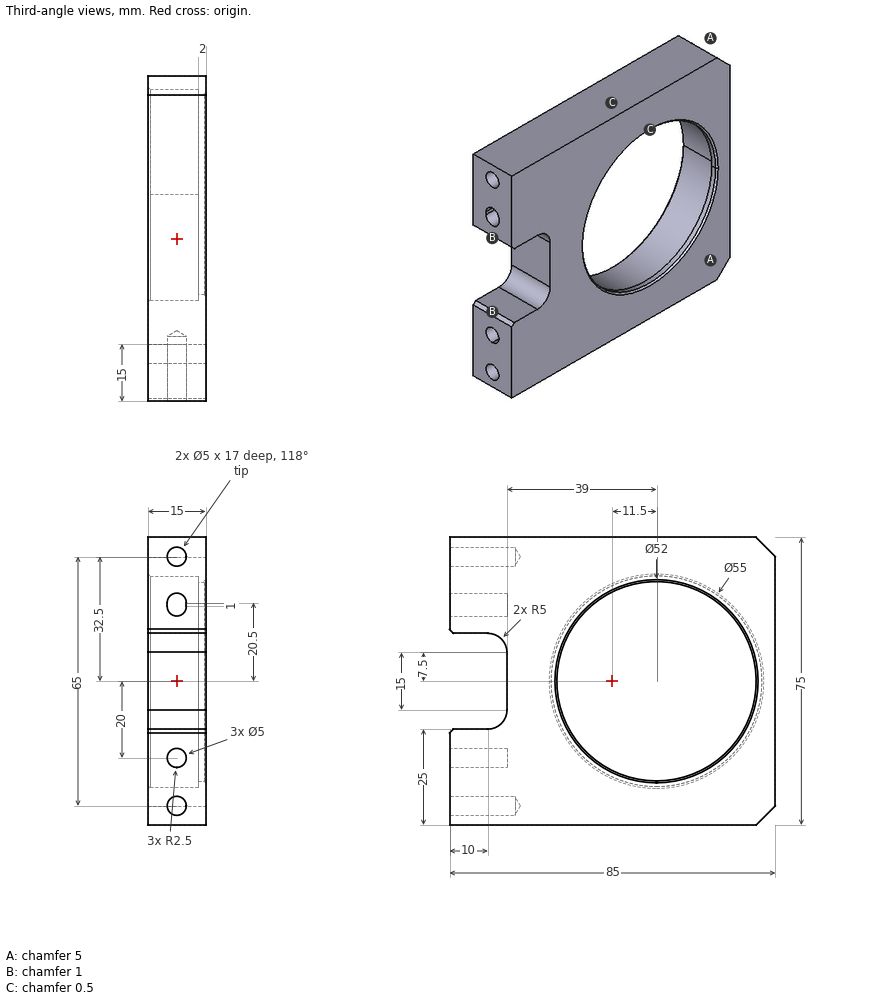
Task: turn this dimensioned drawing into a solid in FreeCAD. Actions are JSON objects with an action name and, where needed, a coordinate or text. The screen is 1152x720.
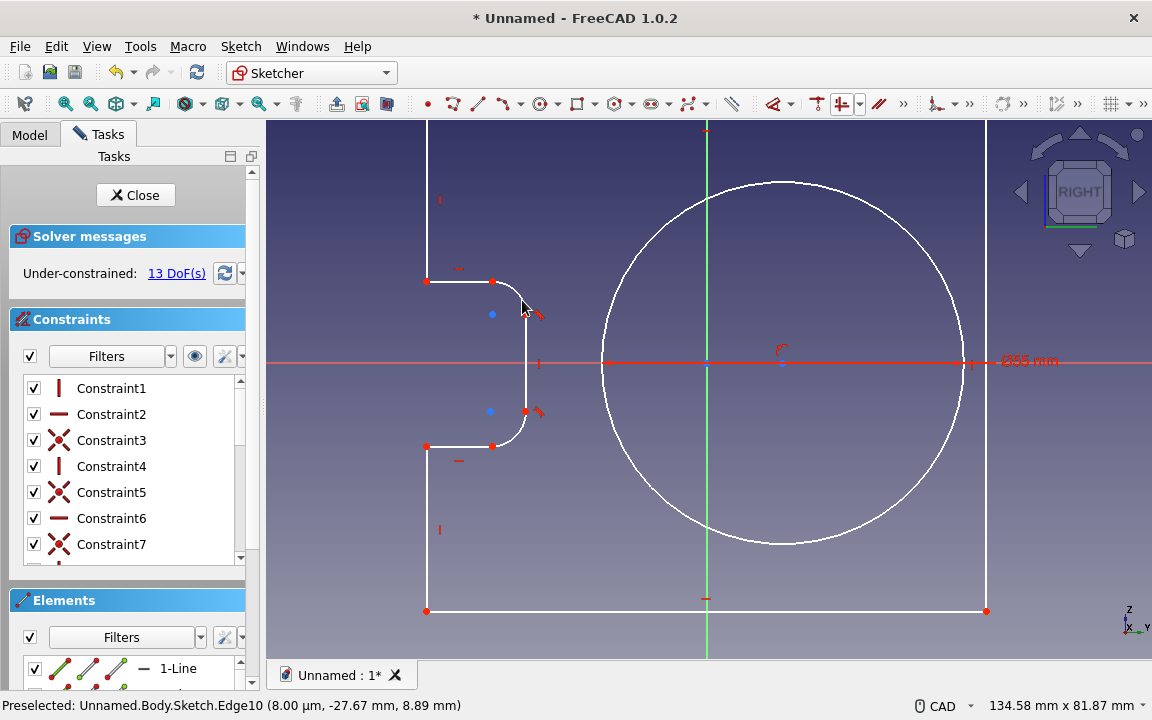
{"action": "left_click", "coordinate": [473, 447]}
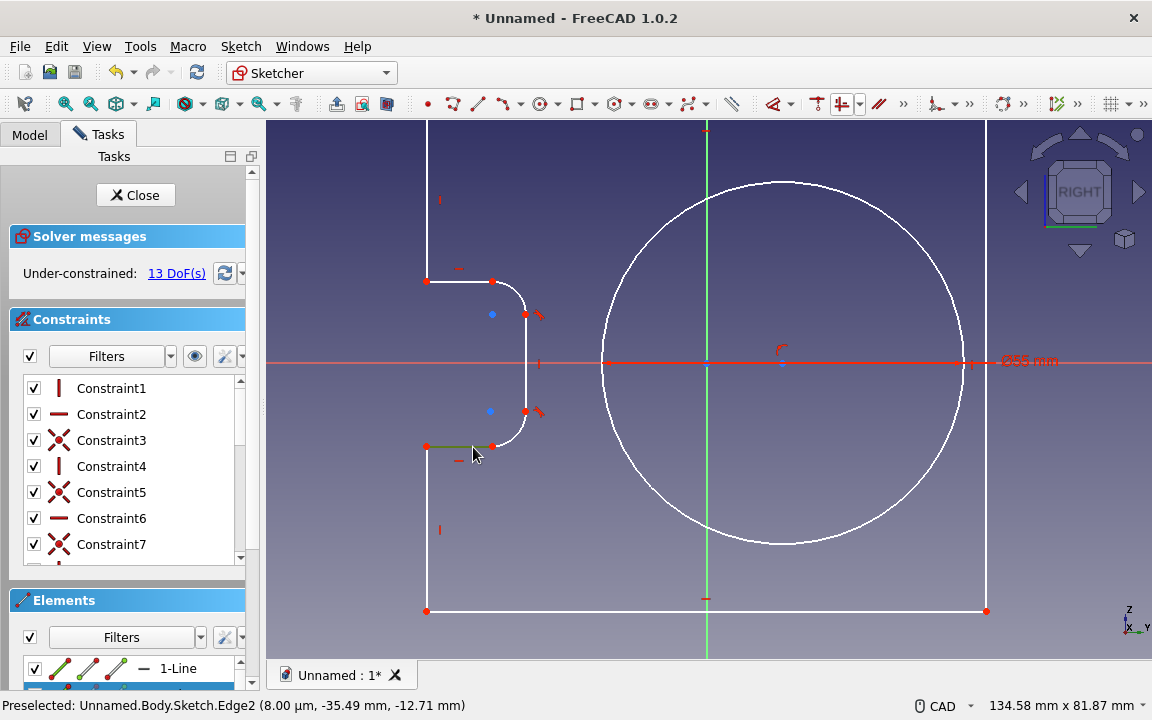
{"action": "left_click", "coordinate": [508, 442]}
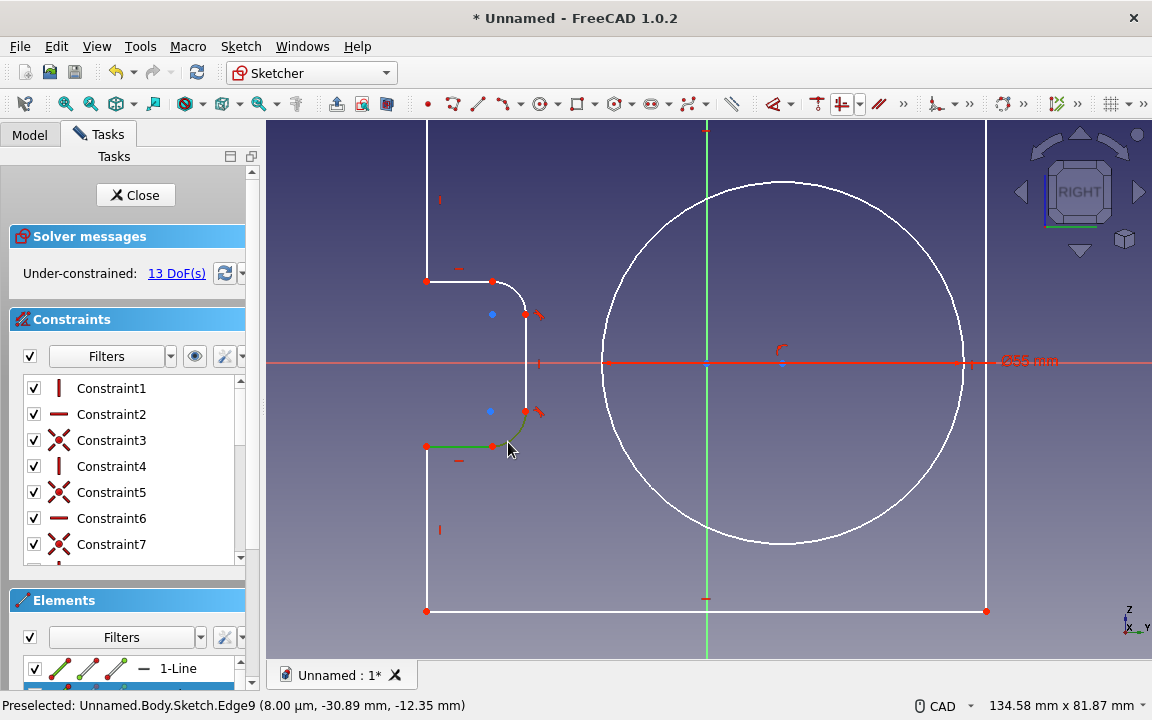
{"action": "key", "text": "t"}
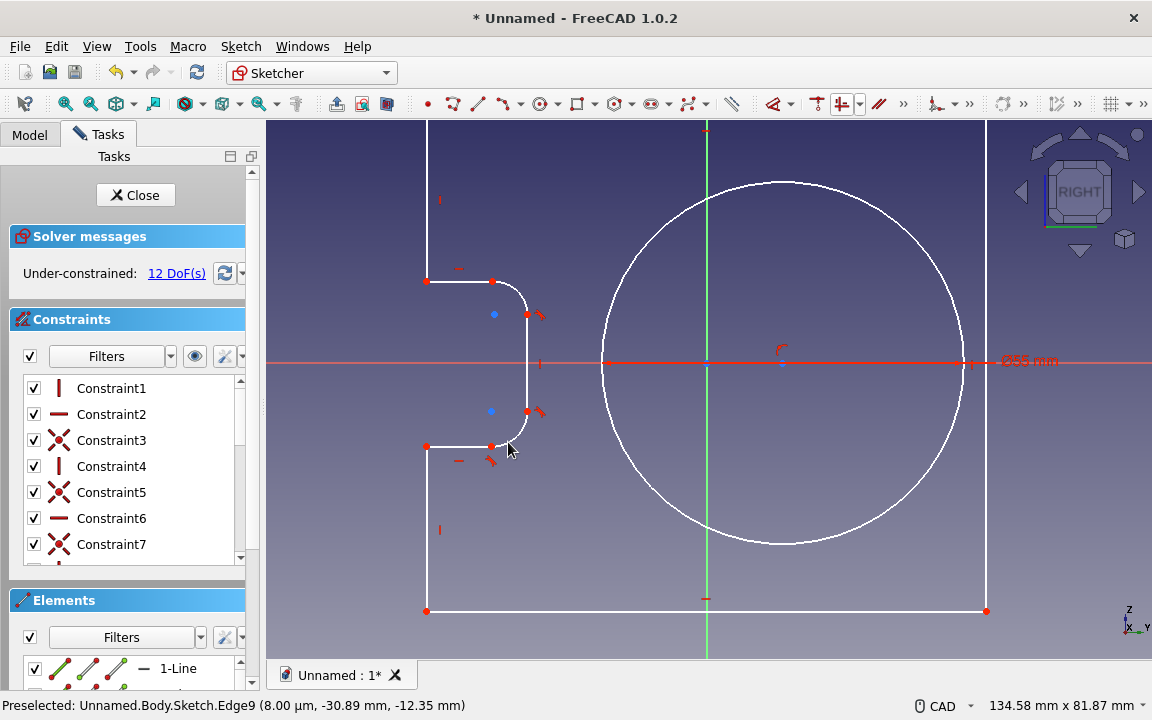
{"action": "left_click", "coordinate": [447, 282]}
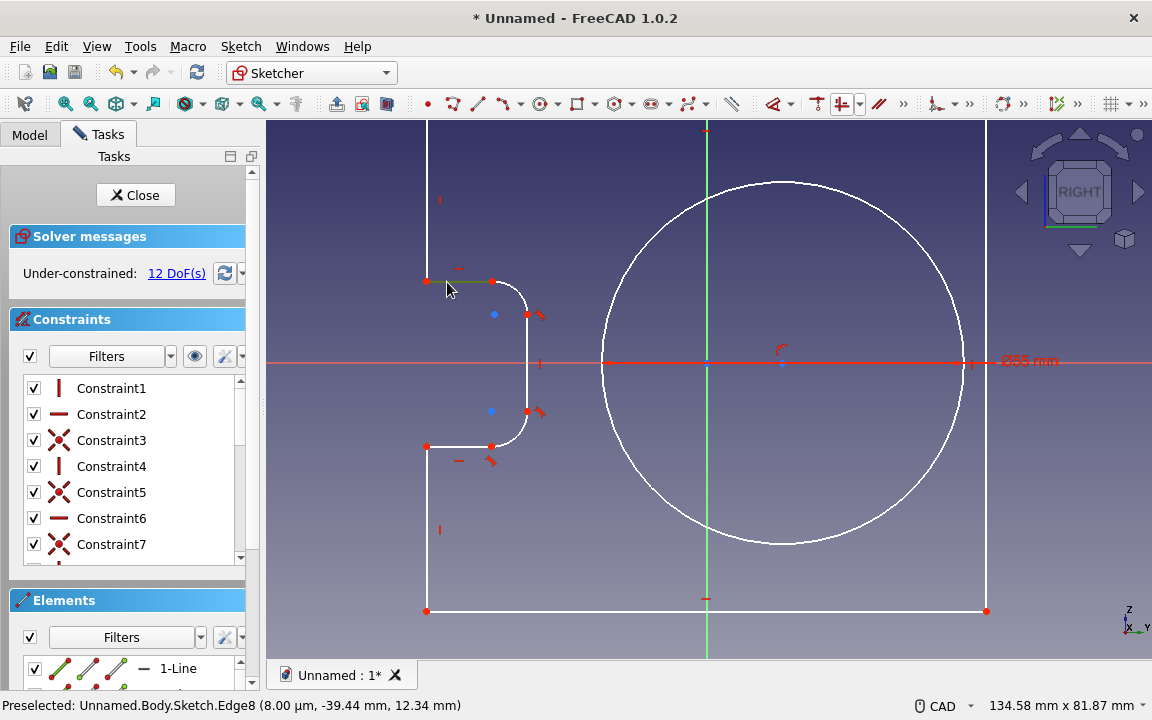
{"action": "left_click", "coordinate": [524, 299]}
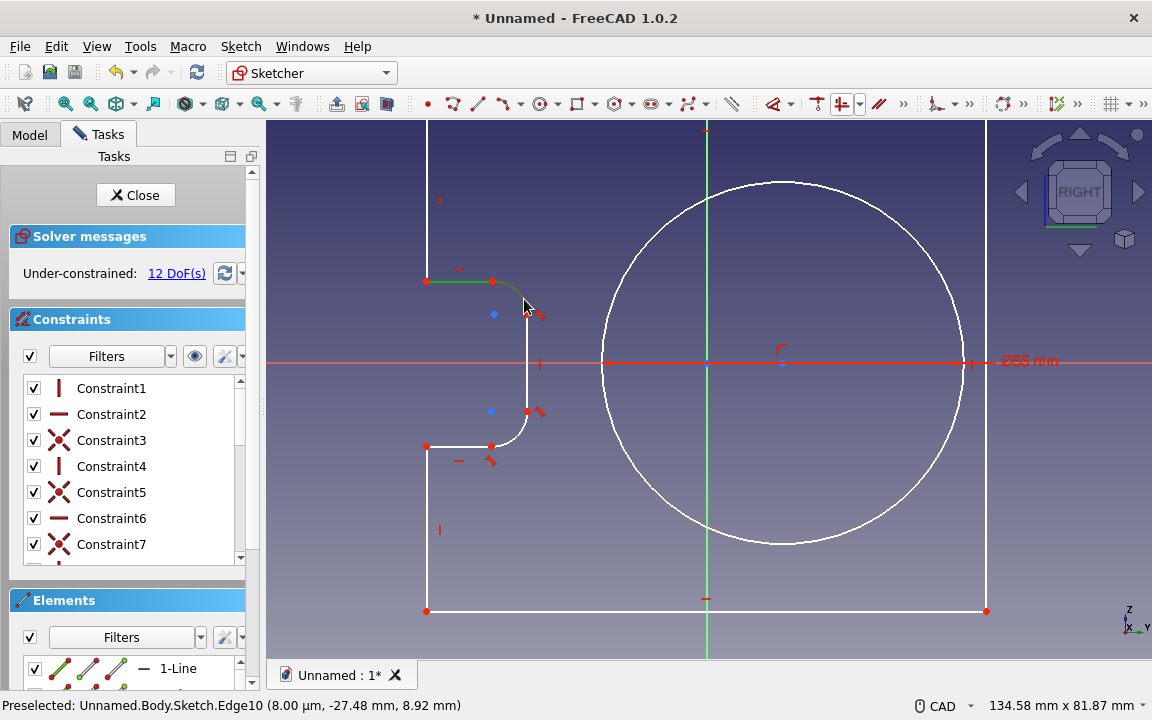
{"action": "key", "text": "t"}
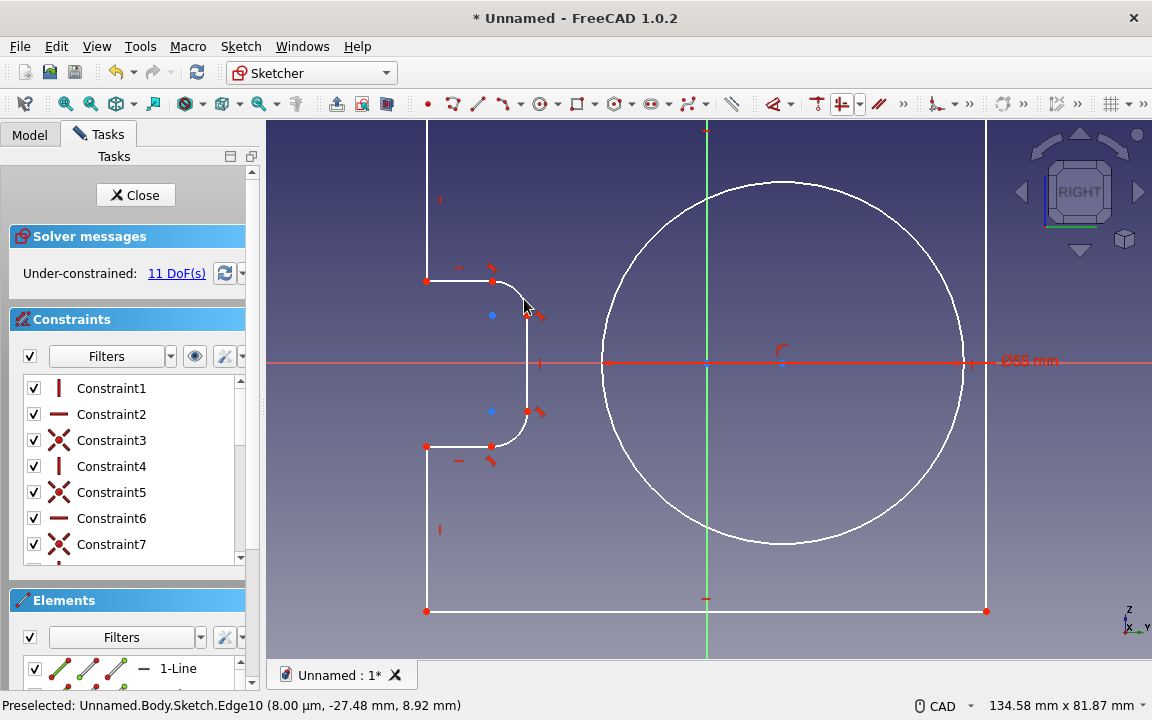
{"action": "left_click", "coordinate": [508, 443]}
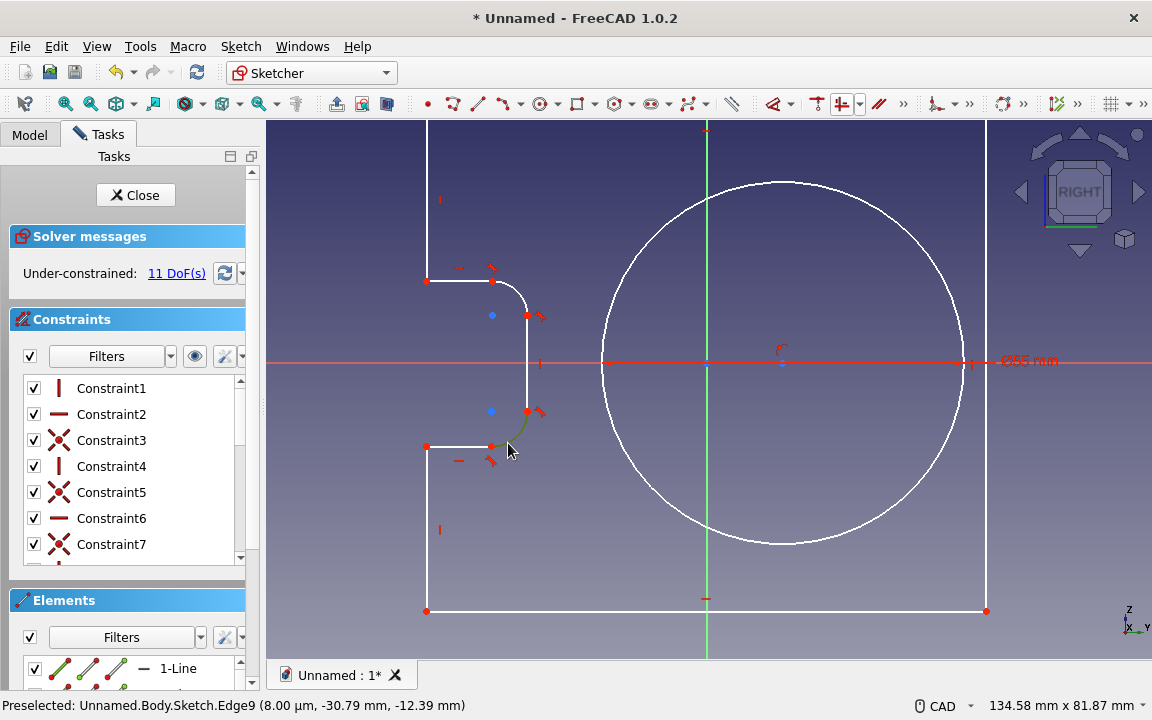
{"action": "left_click", "coordinate": [524, 300]}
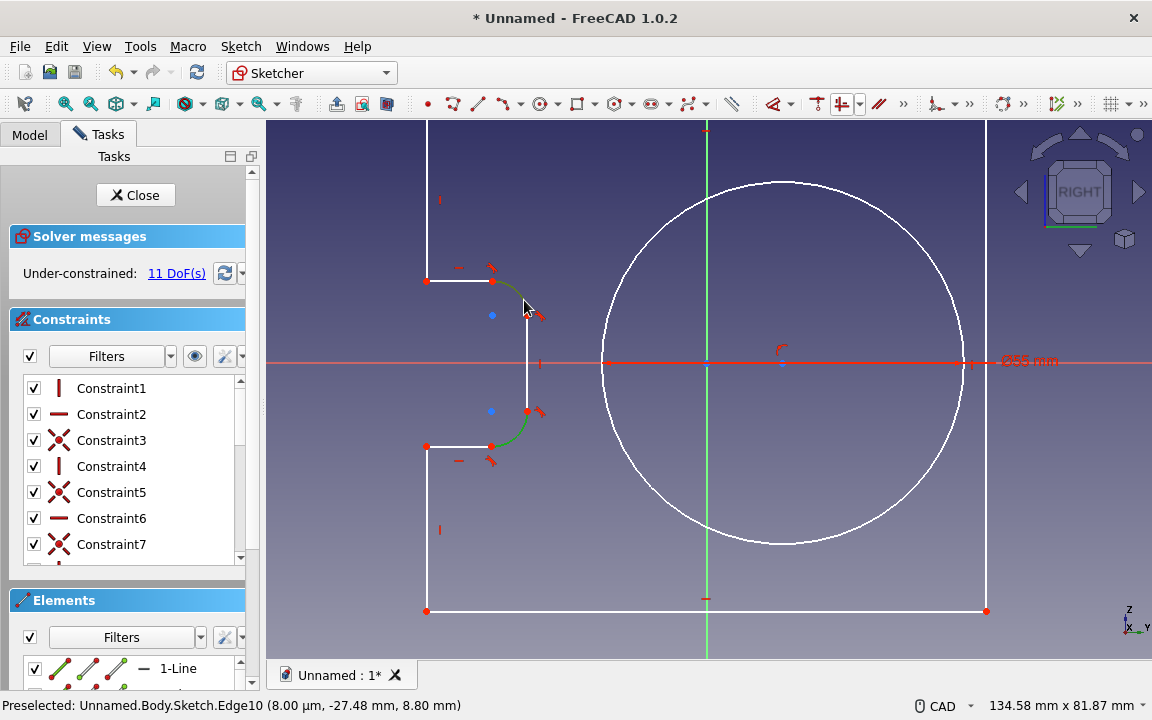
{"action": "key", "text": "e"}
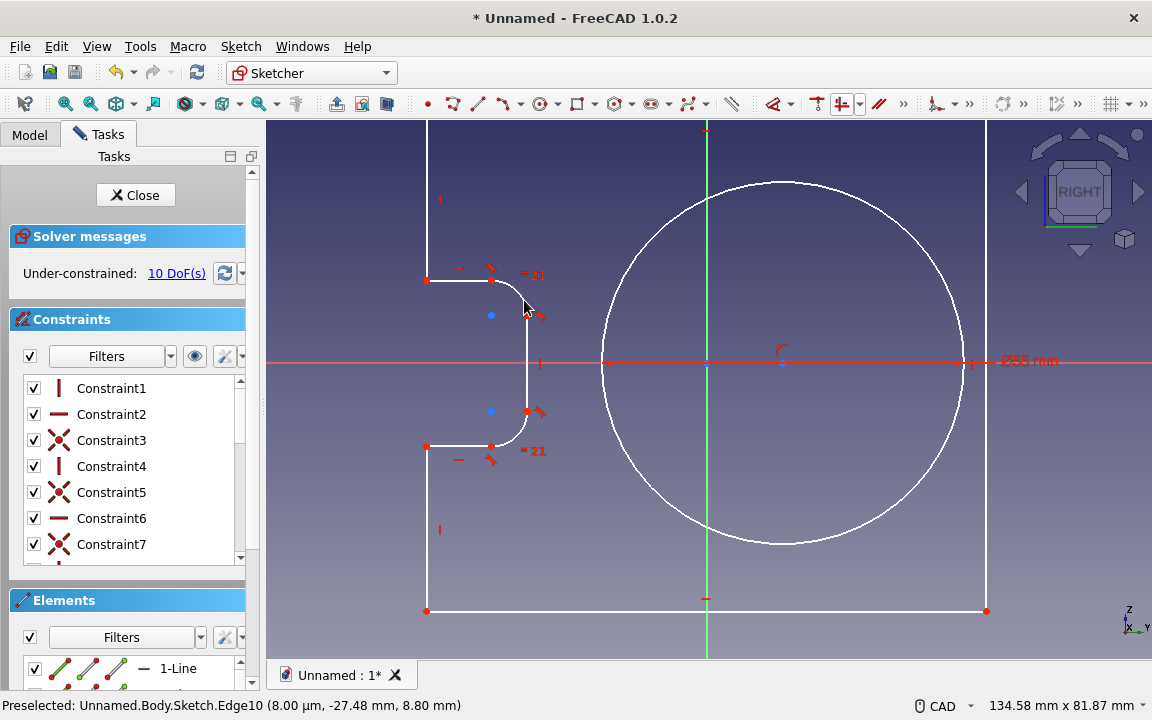
{"action": "left_click", "coordinate": [772, 104]}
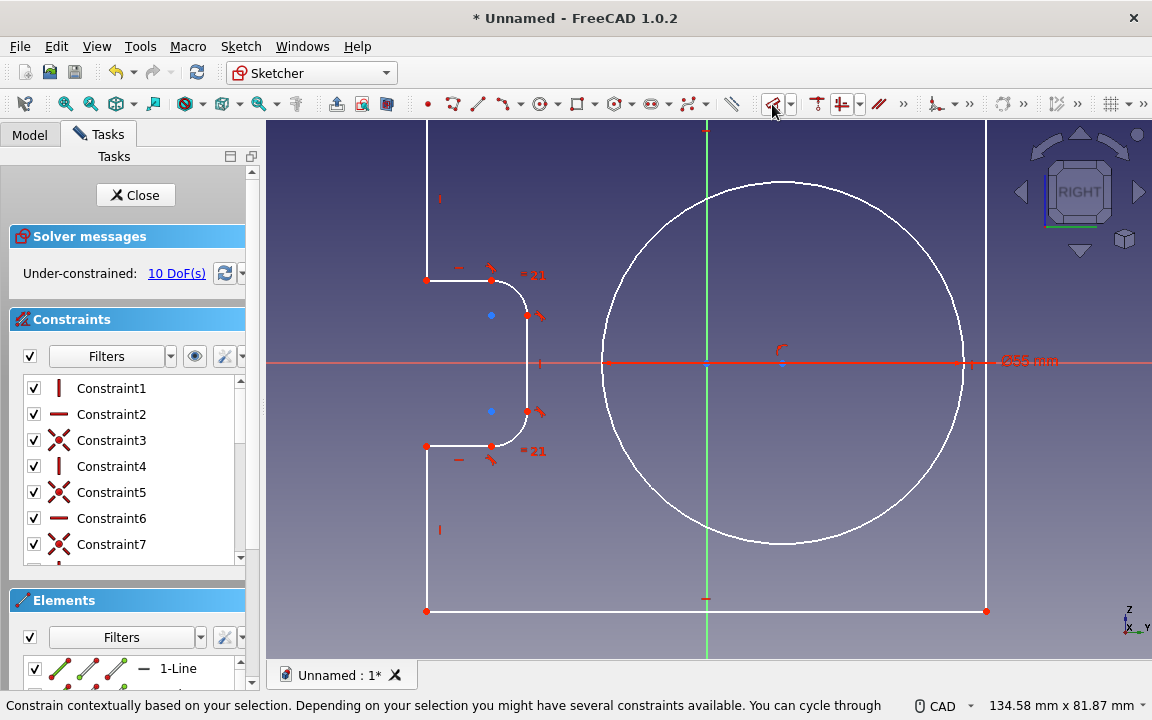
{"action": "left_click", "coordinate": [508, 443]}
{"action": "left_click", "coordinate": [522, 472]}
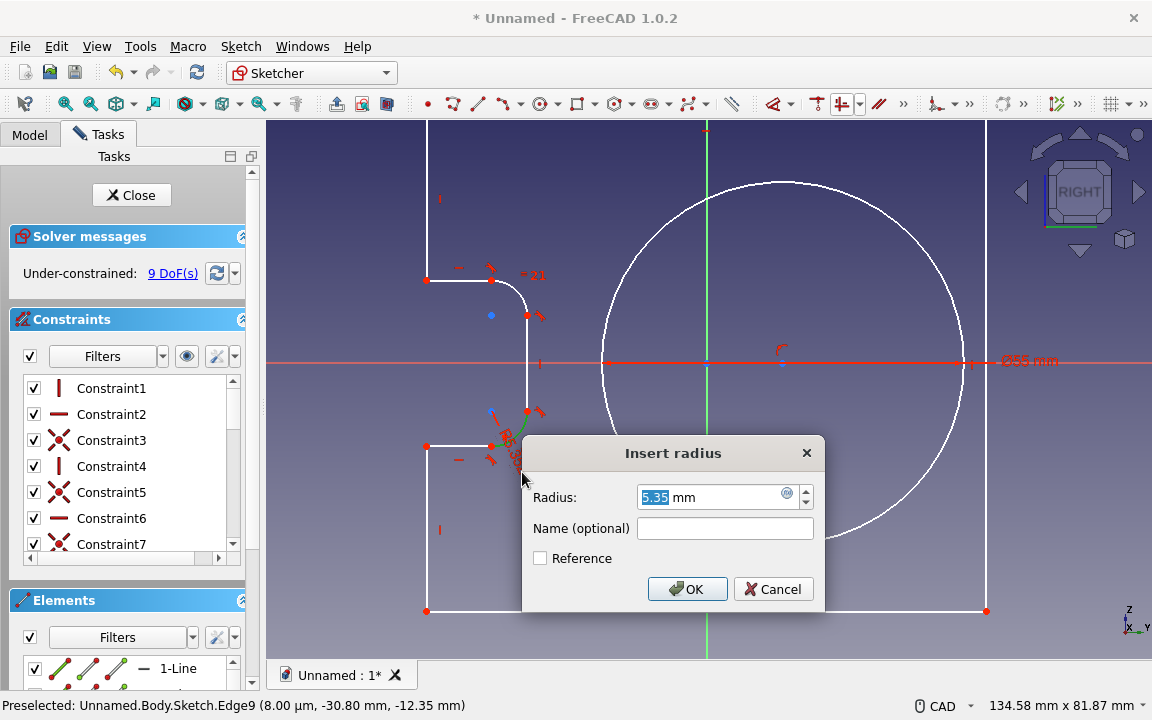
{"action": "type", "text": "5"}
{"action": "key", "text": "Return"}